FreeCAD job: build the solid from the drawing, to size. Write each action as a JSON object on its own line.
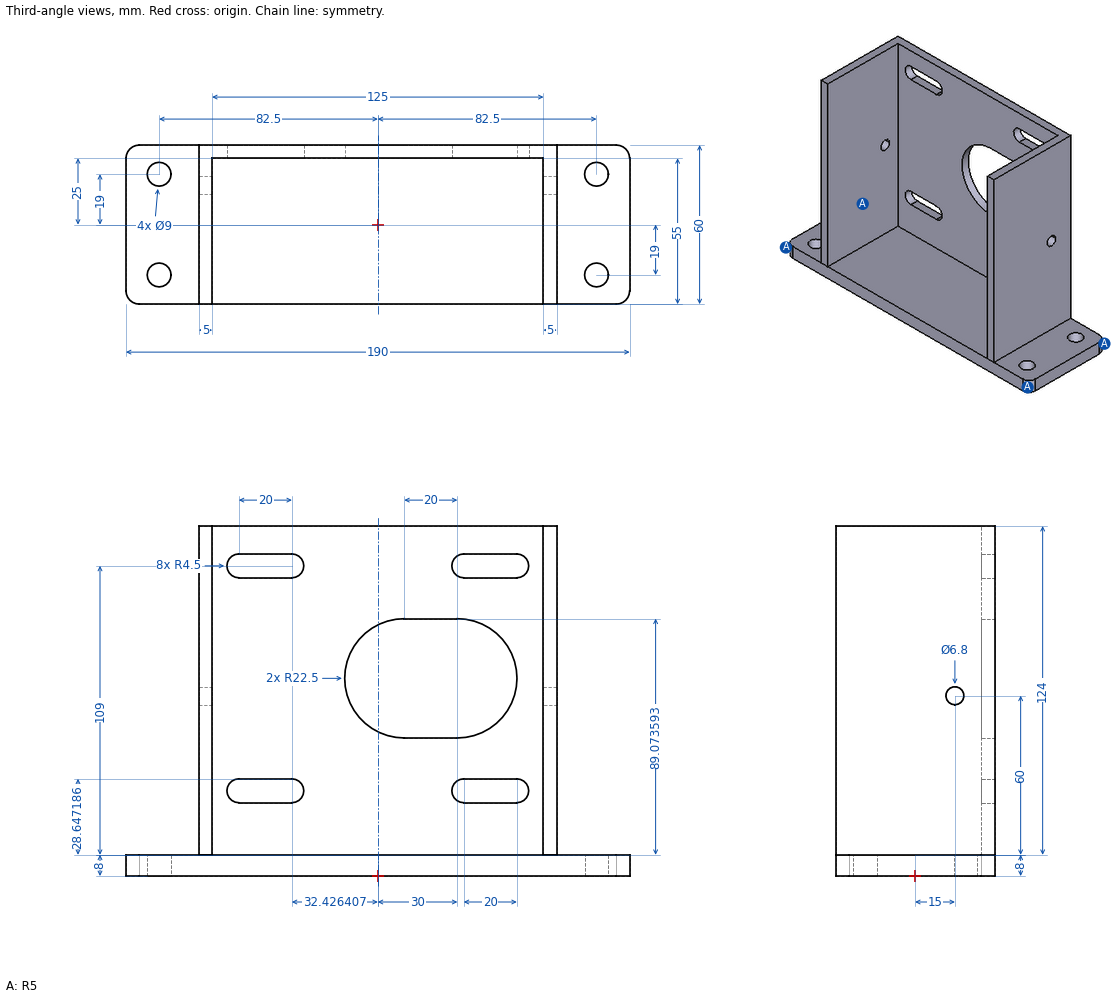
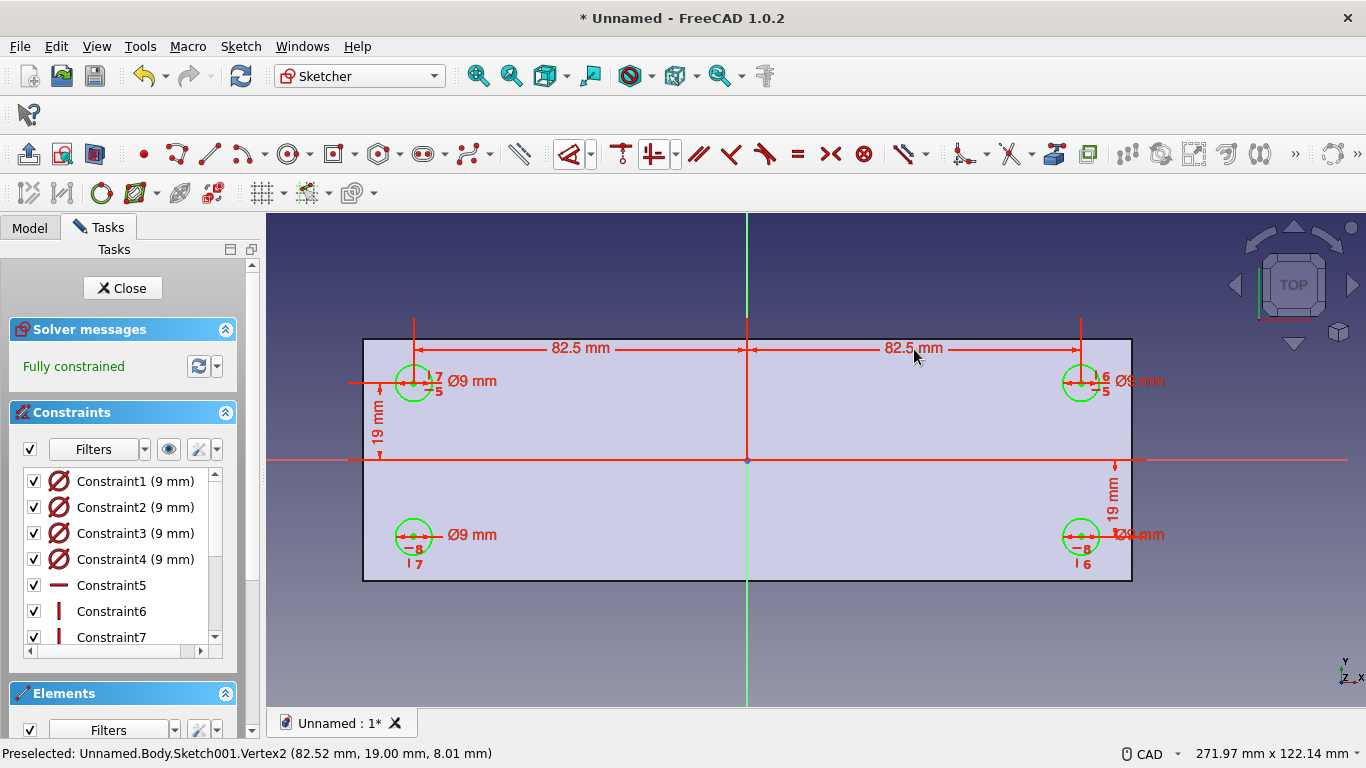
{"action": "left_click", "coordinate": [123, 288]}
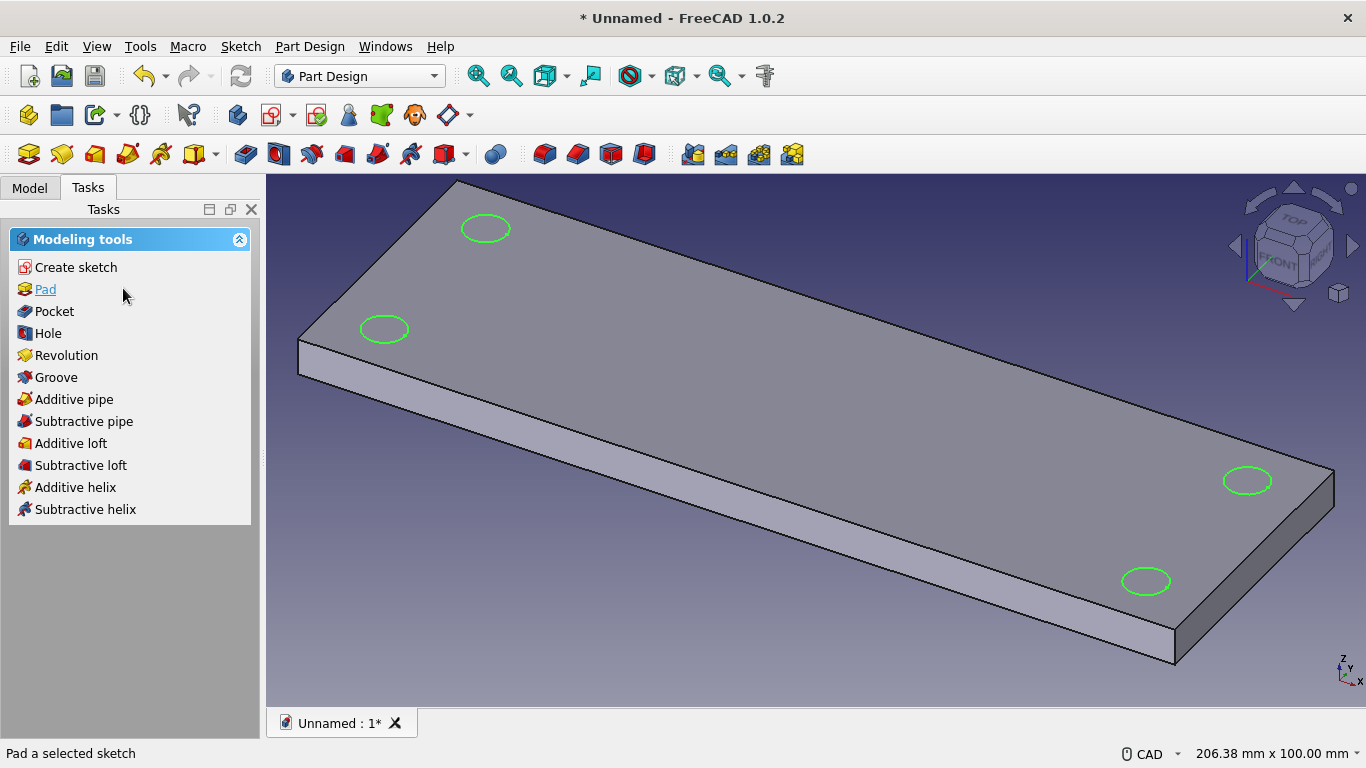
{"action": "left_click", "coordinate": [246, 154]}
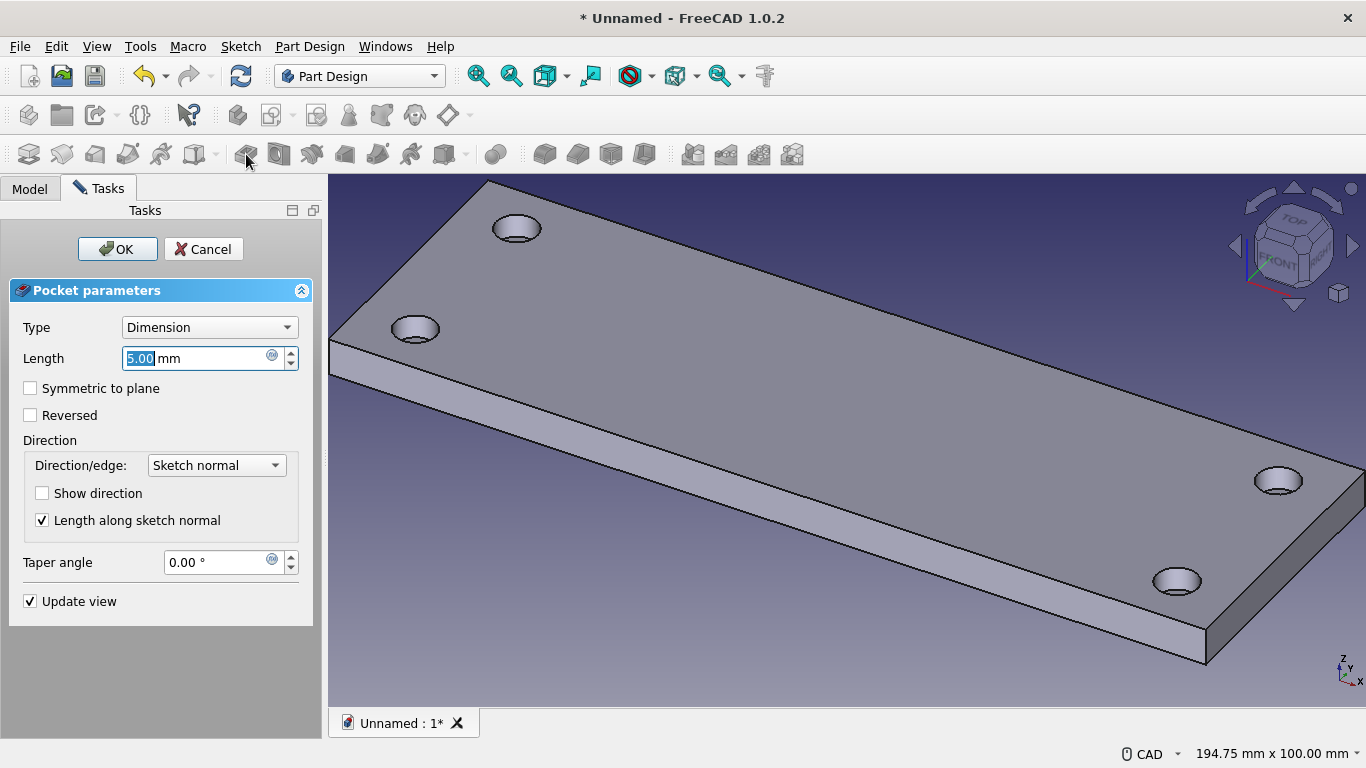
{"action": "type", "text": "8"}
{"action": "key", "text": "Tab"}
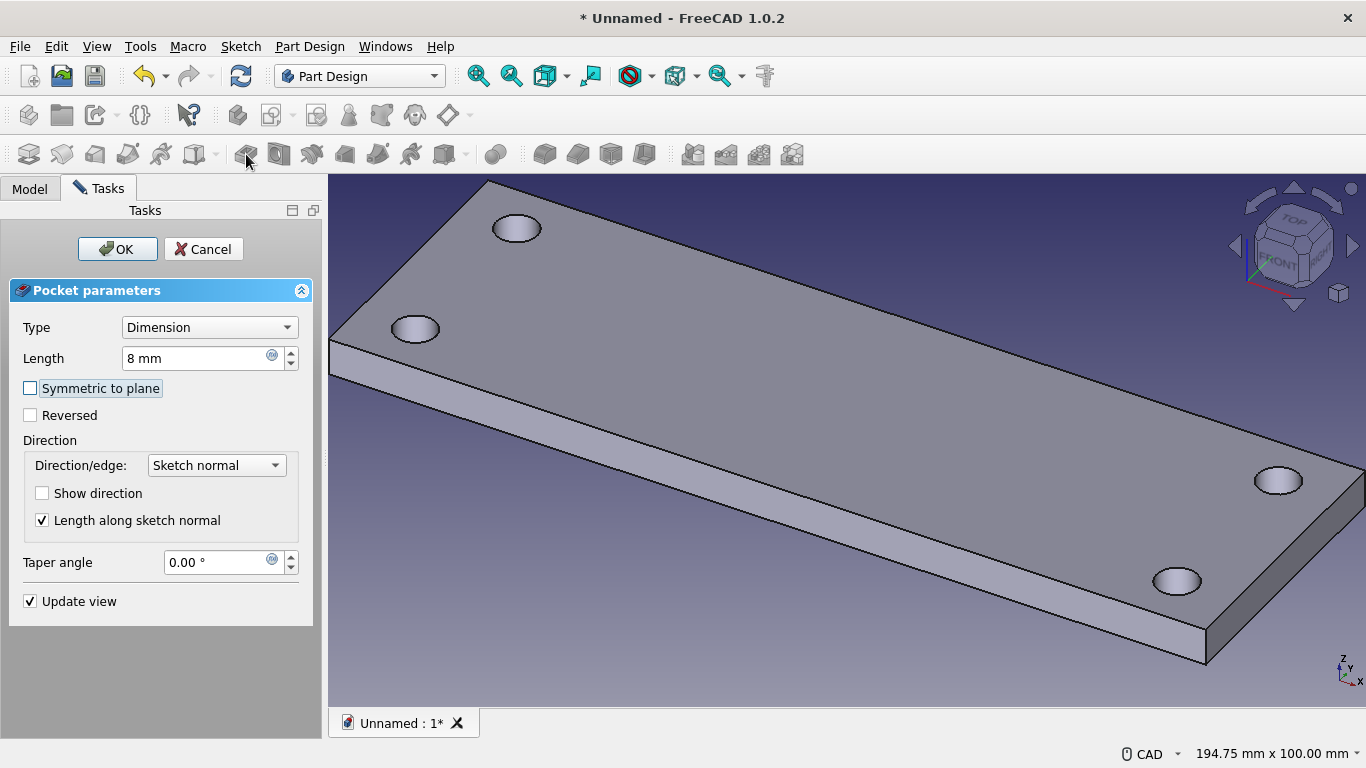
{"action": "left_click", "coordinate": [118, 249]}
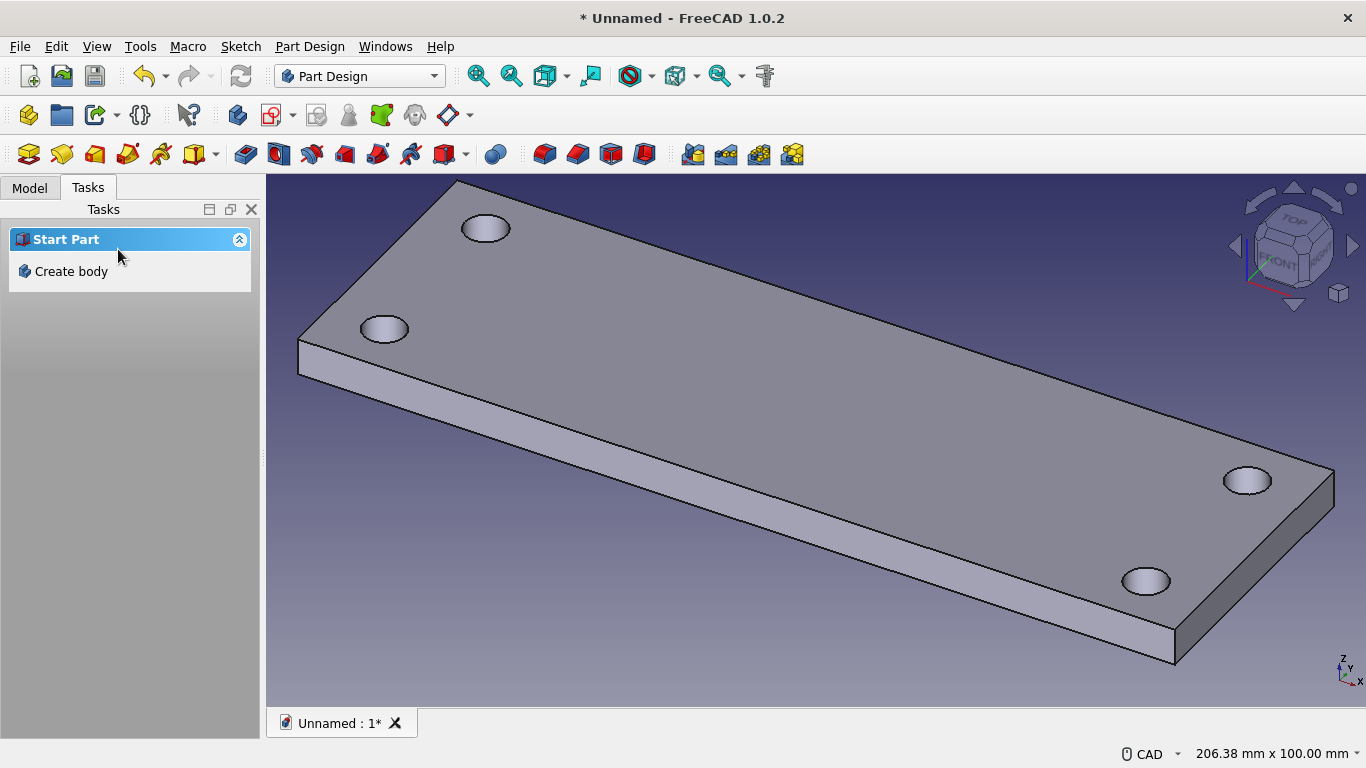
{"action": "left_click", "coordinate": [1175, 646]}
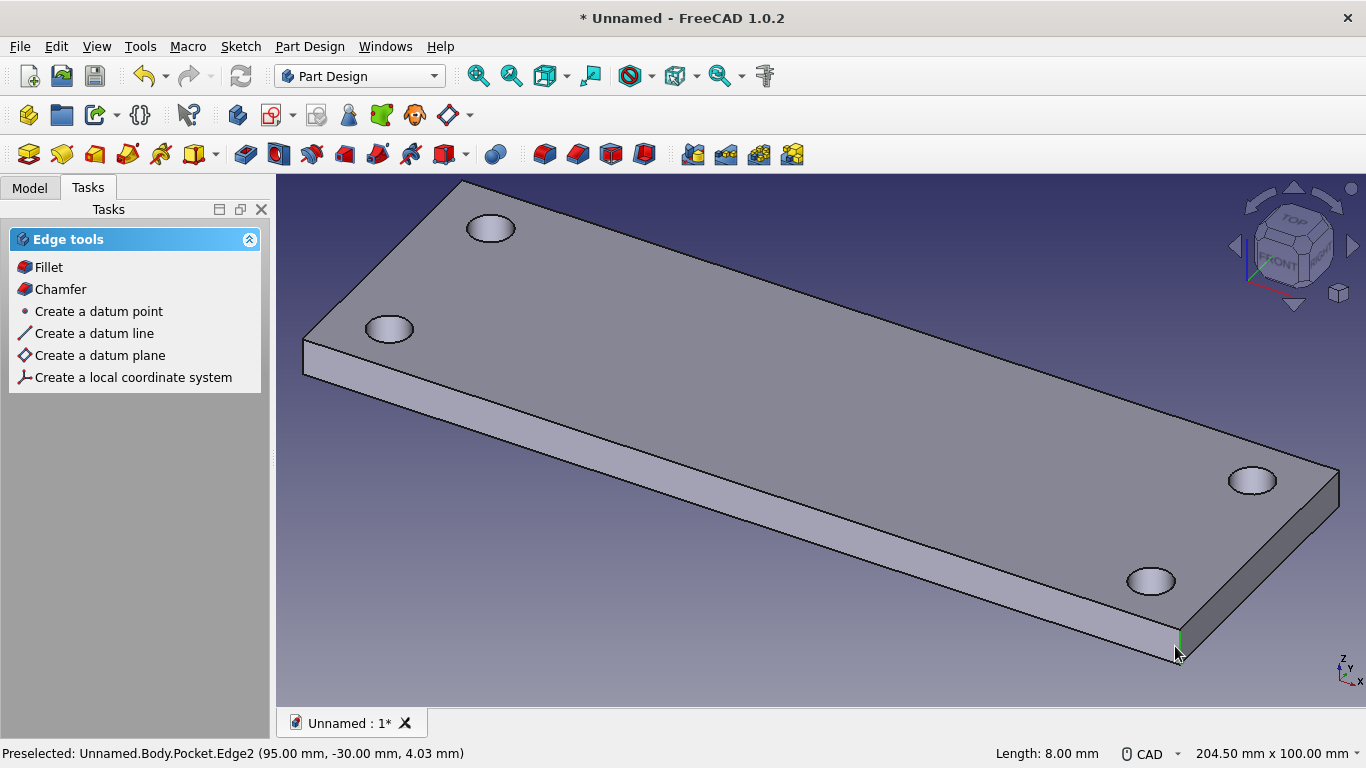
{"action": "key", "text": "0"}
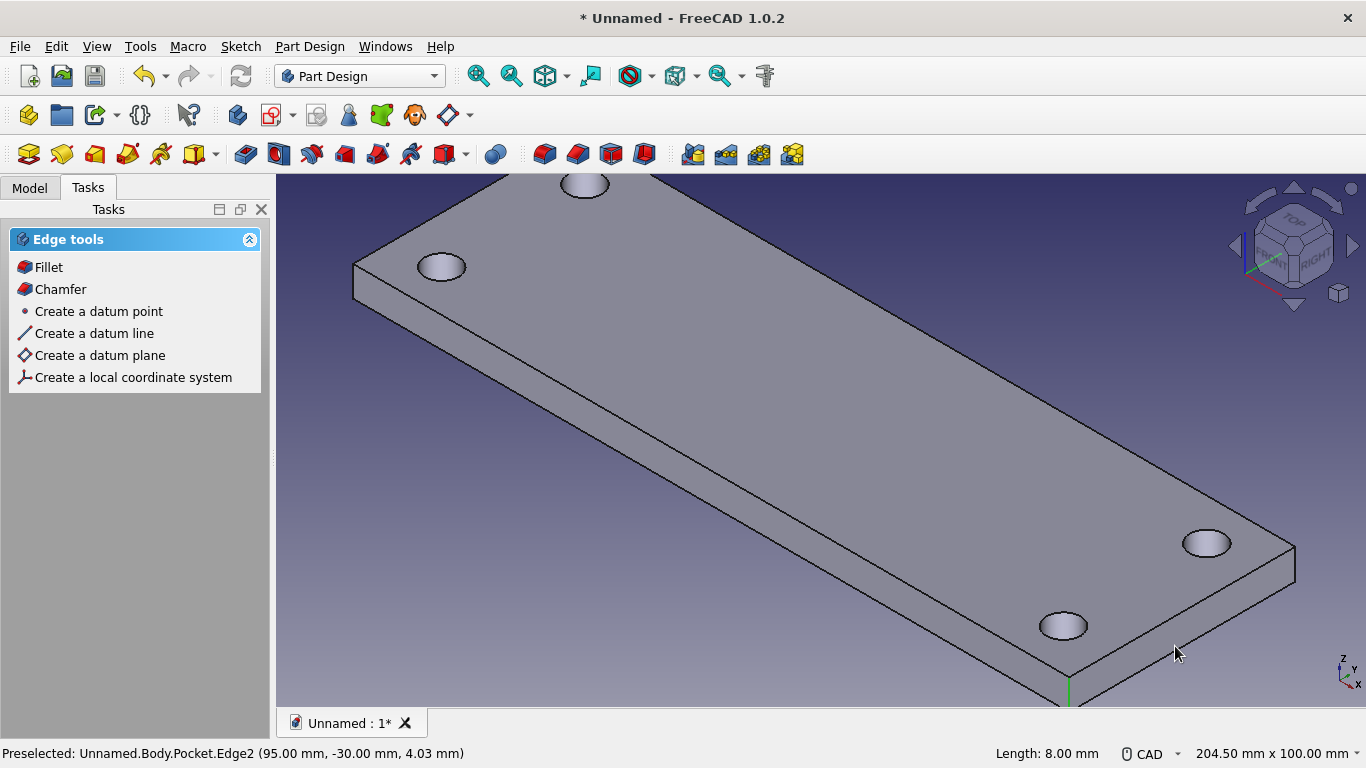
{"action": "left_click", "coordinate": [479, 76]}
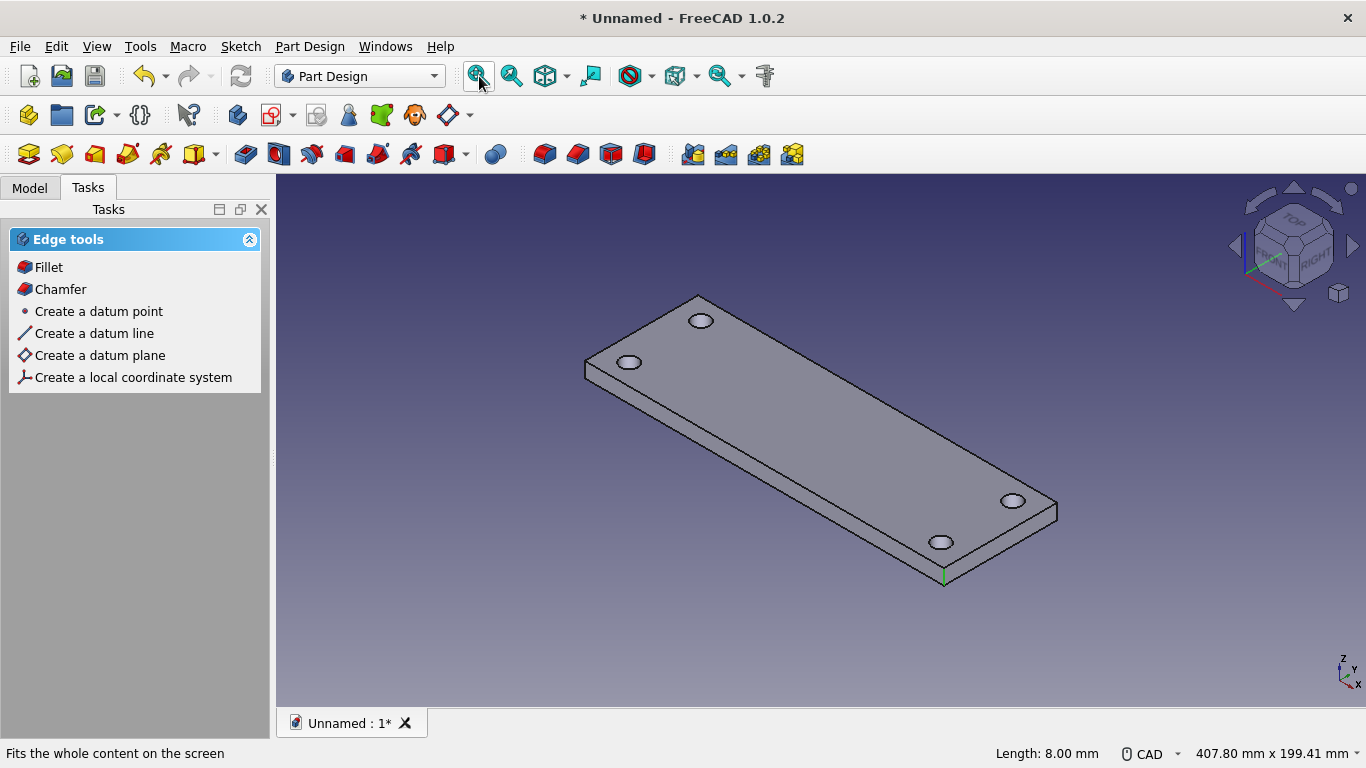
{"action": "scroll", "coordinate": [585, 369], "scroll_direction": "up", "scroll_amount": 4}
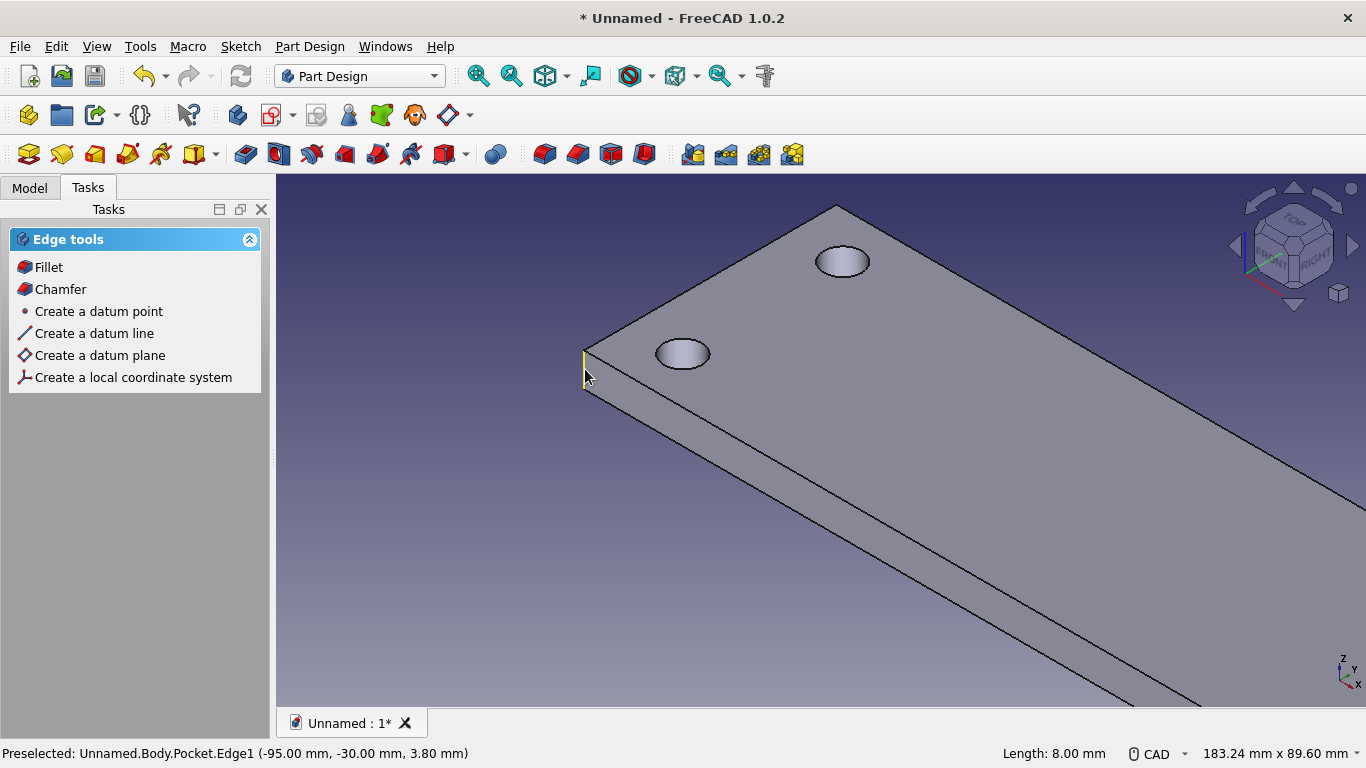
{"action": "left_click", "coordinate": [479, 76]}